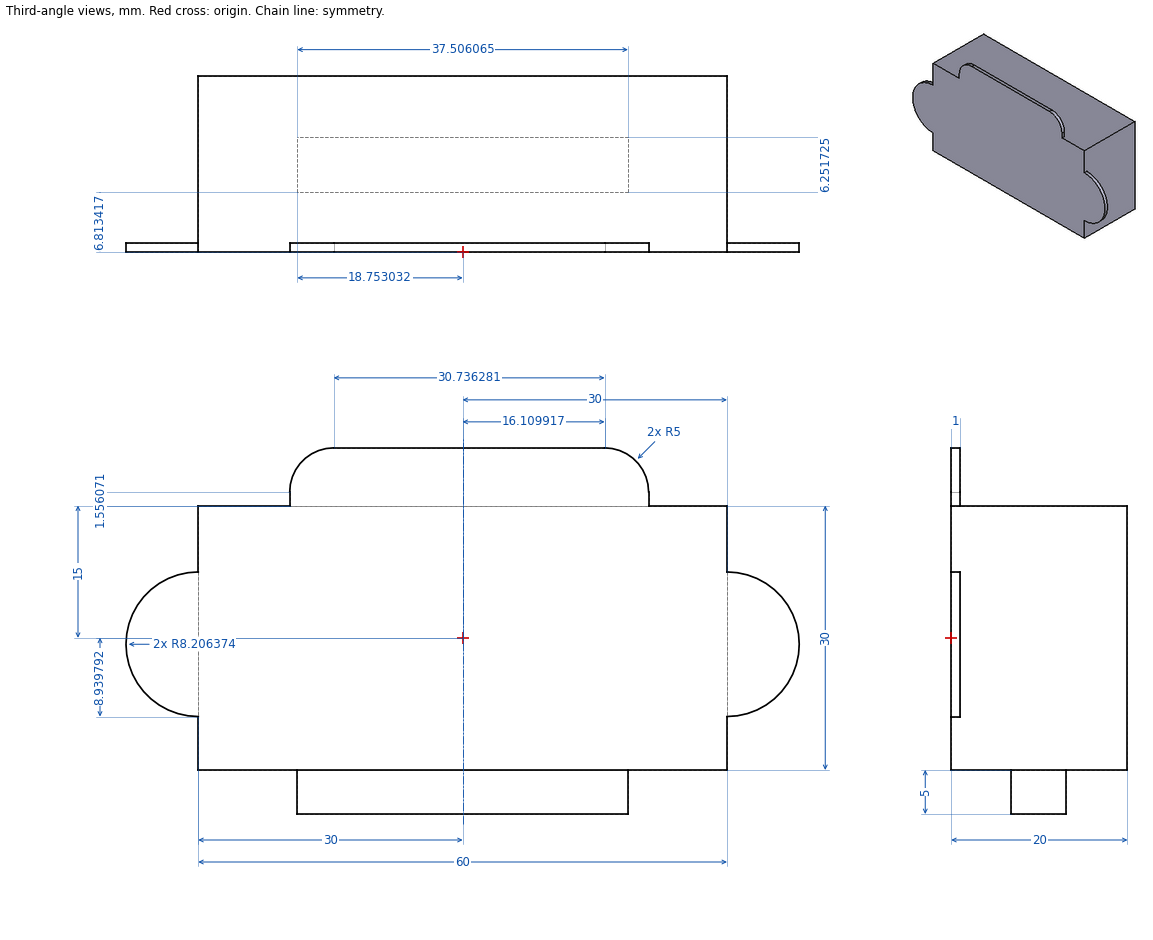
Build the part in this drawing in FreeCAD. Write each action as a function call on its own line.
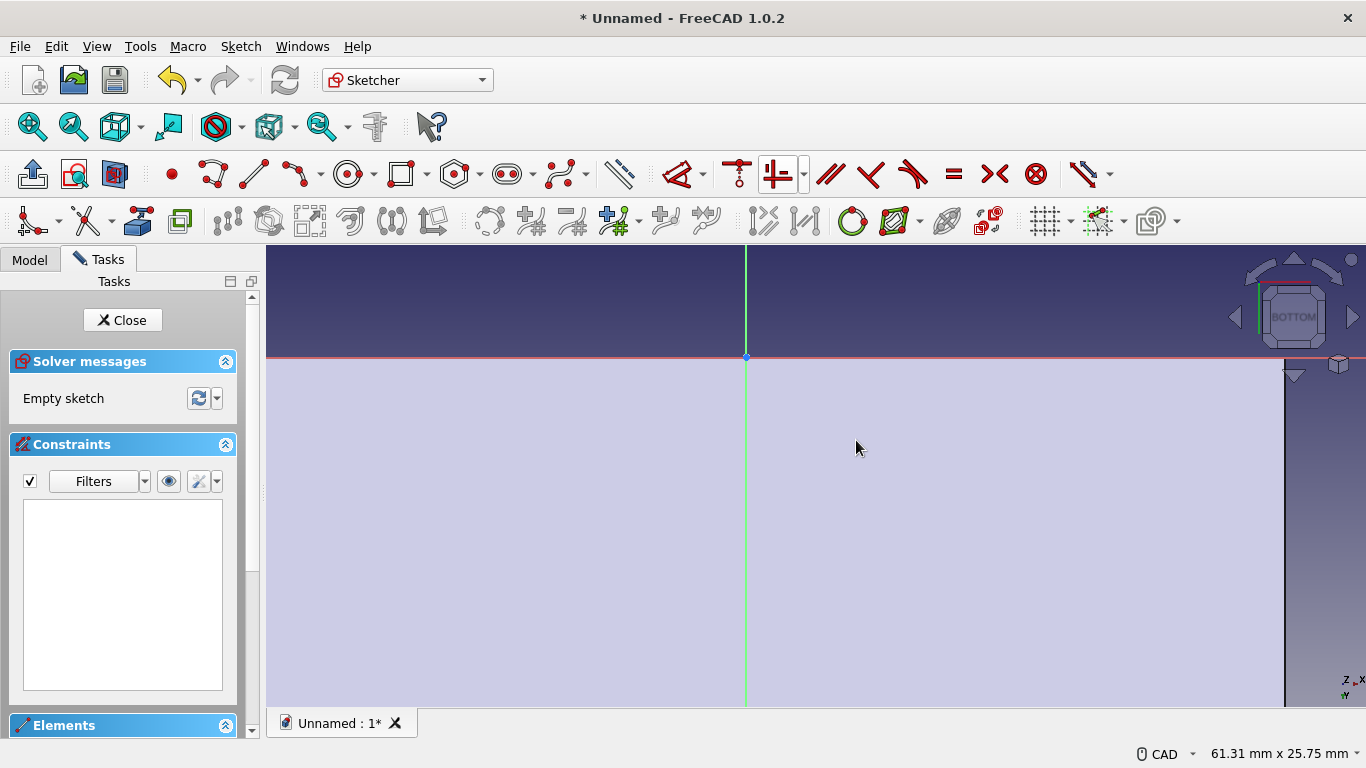
key(g)
key(r)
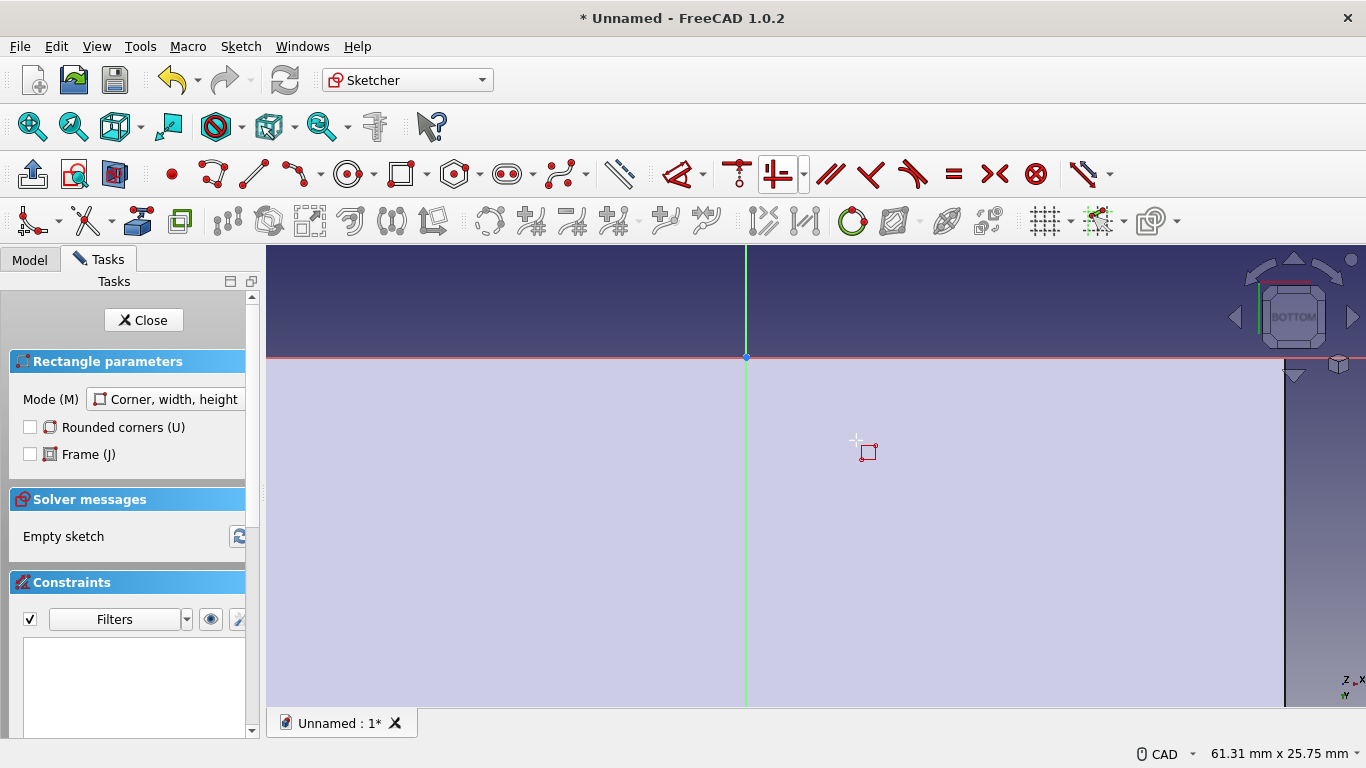
click(410, 480)
move(1083, 592)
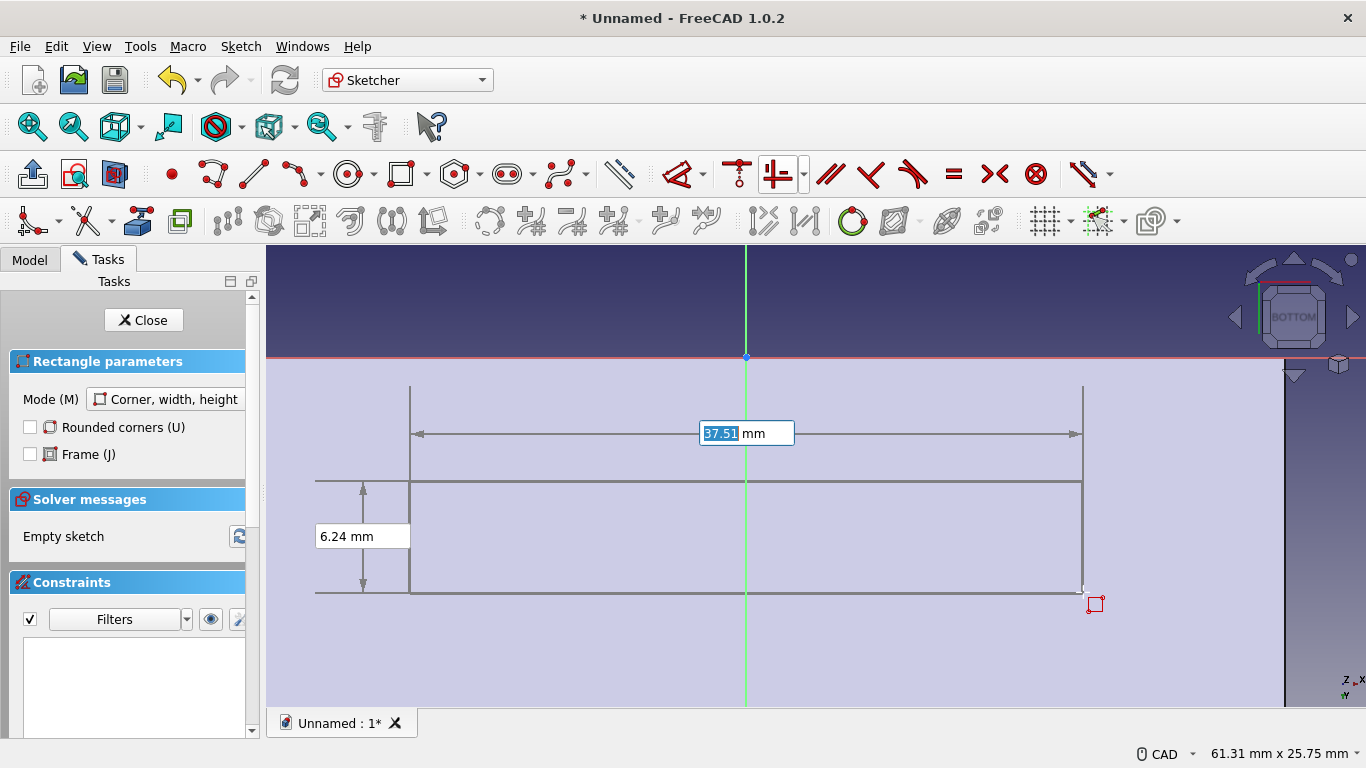
text(37.506065)
key(Tab)
text(6.251725)
key(Return)
key(Escape)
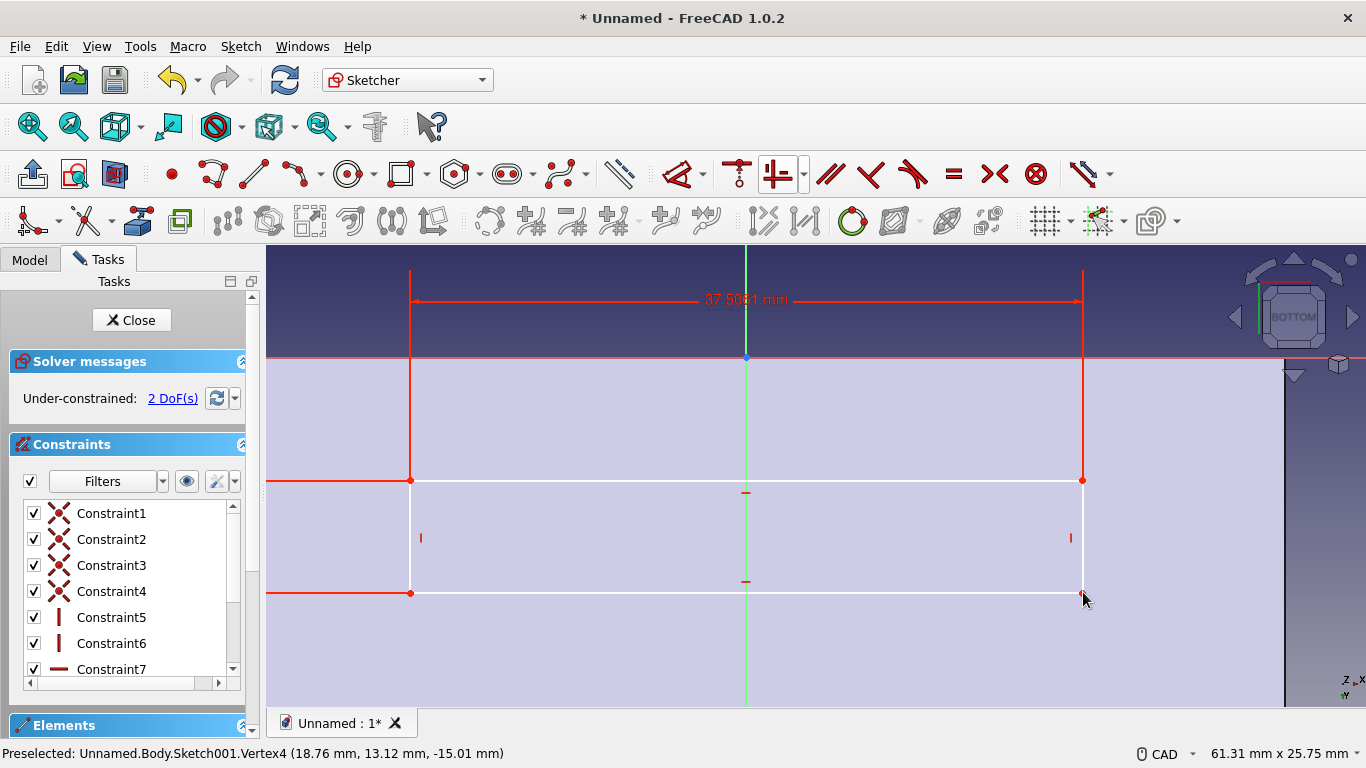
key(d)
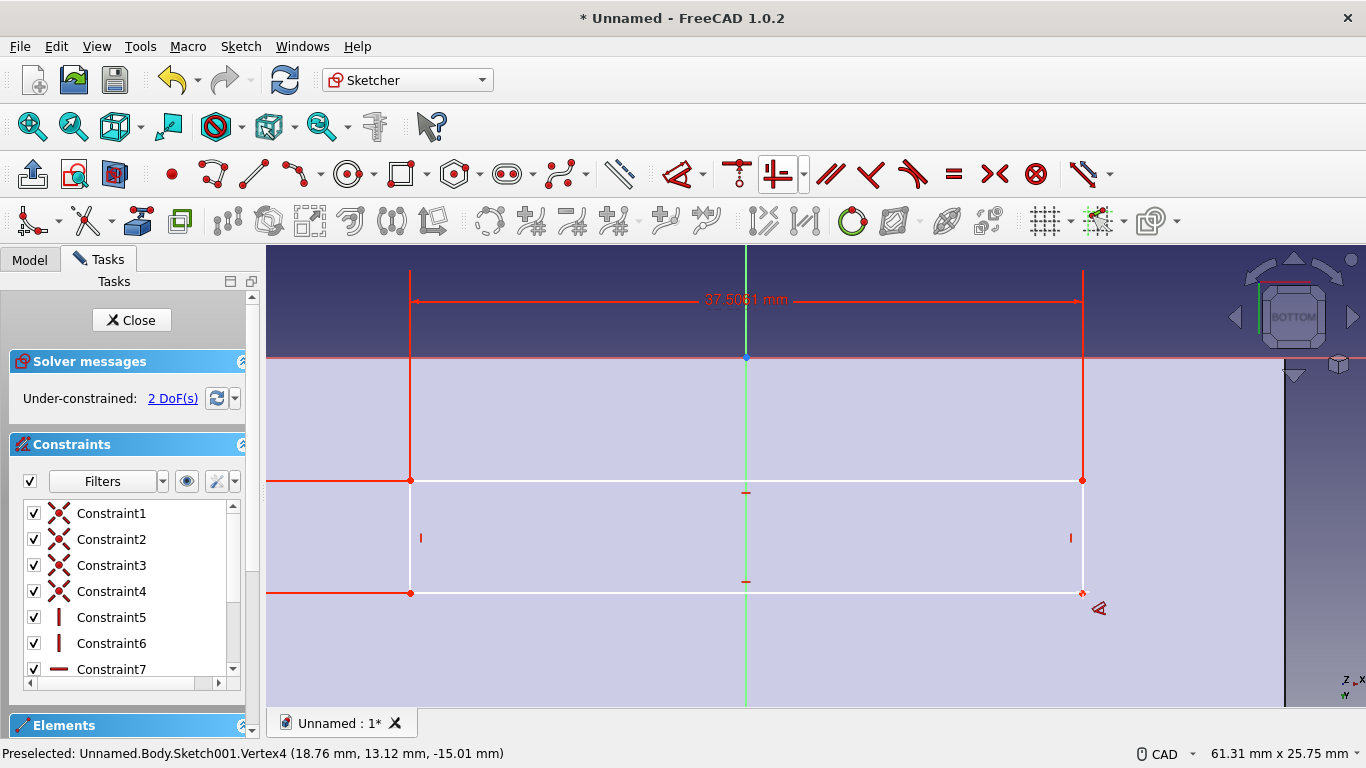
click(410, 481)
click(376, 419)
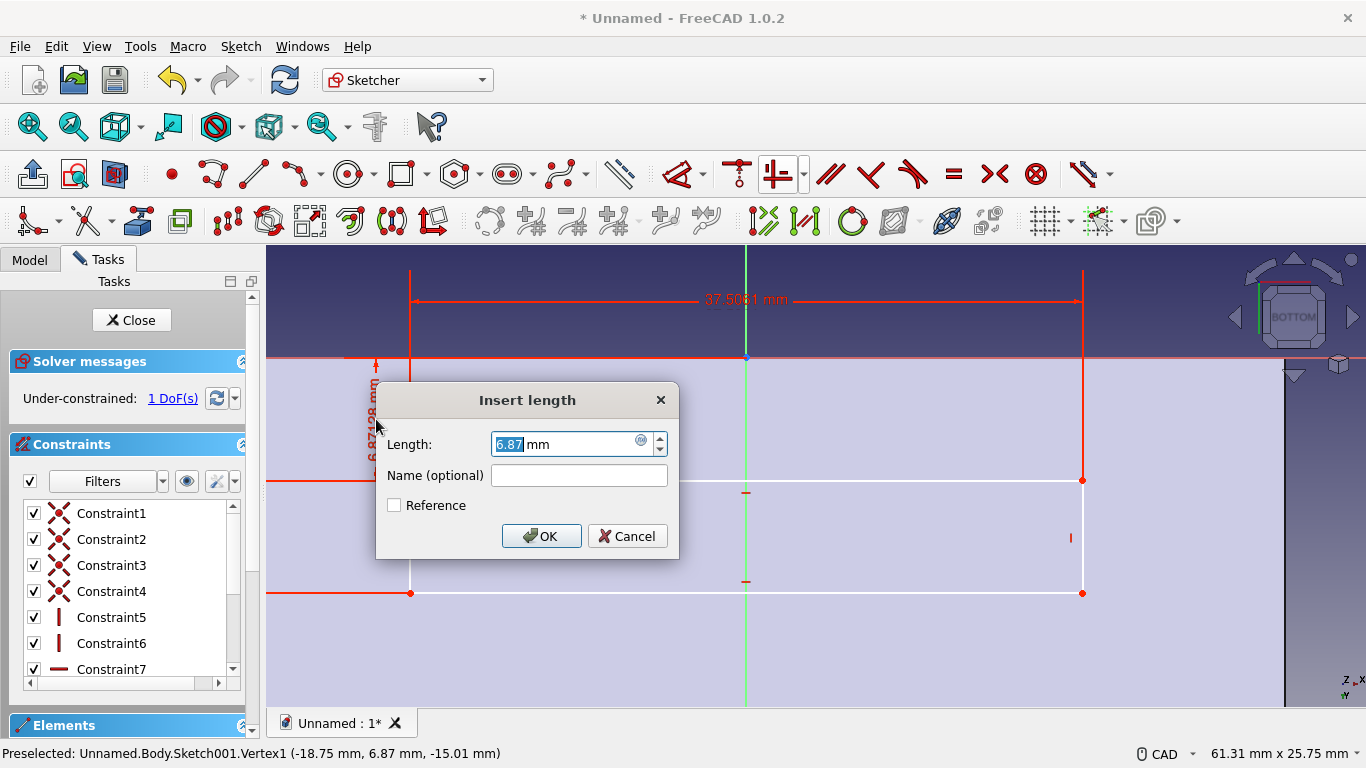
text(6.813417)
key(Return)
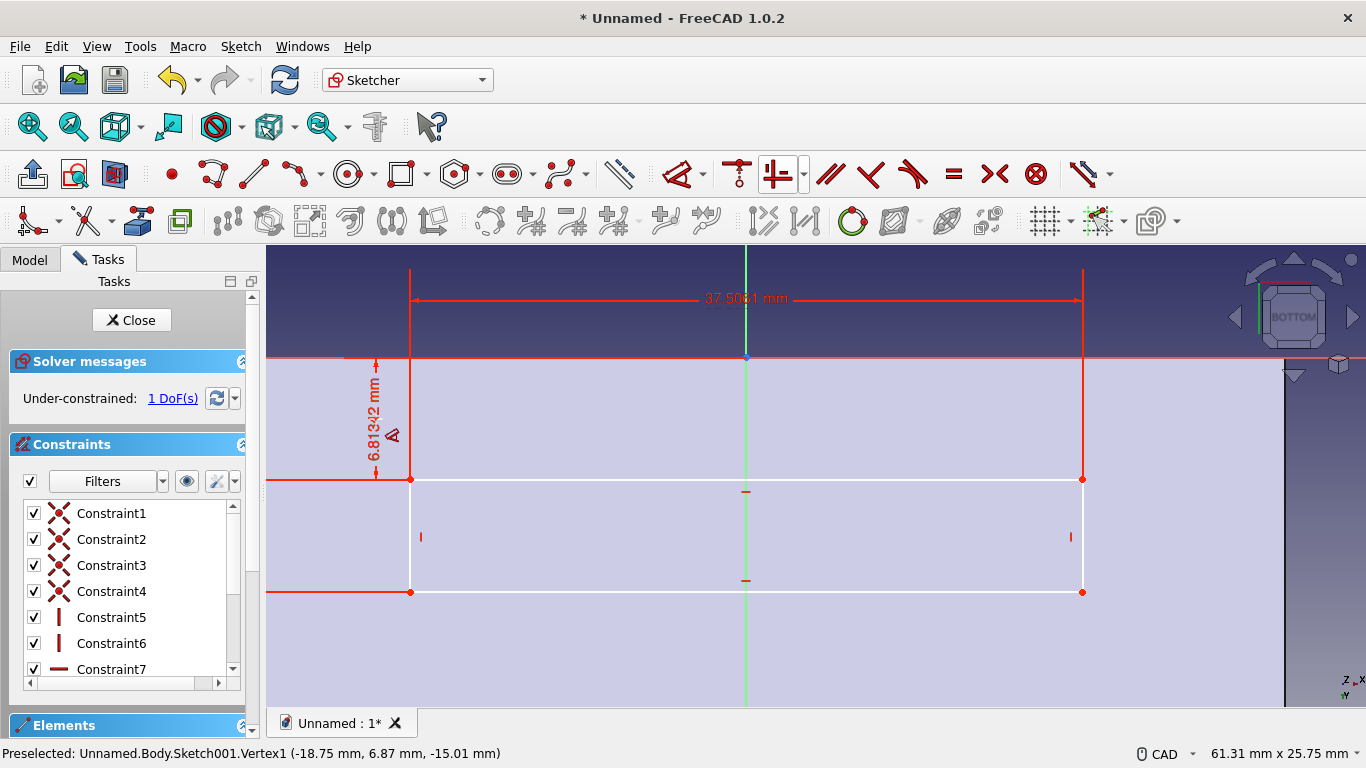
click(410, 480)
click(578, 324)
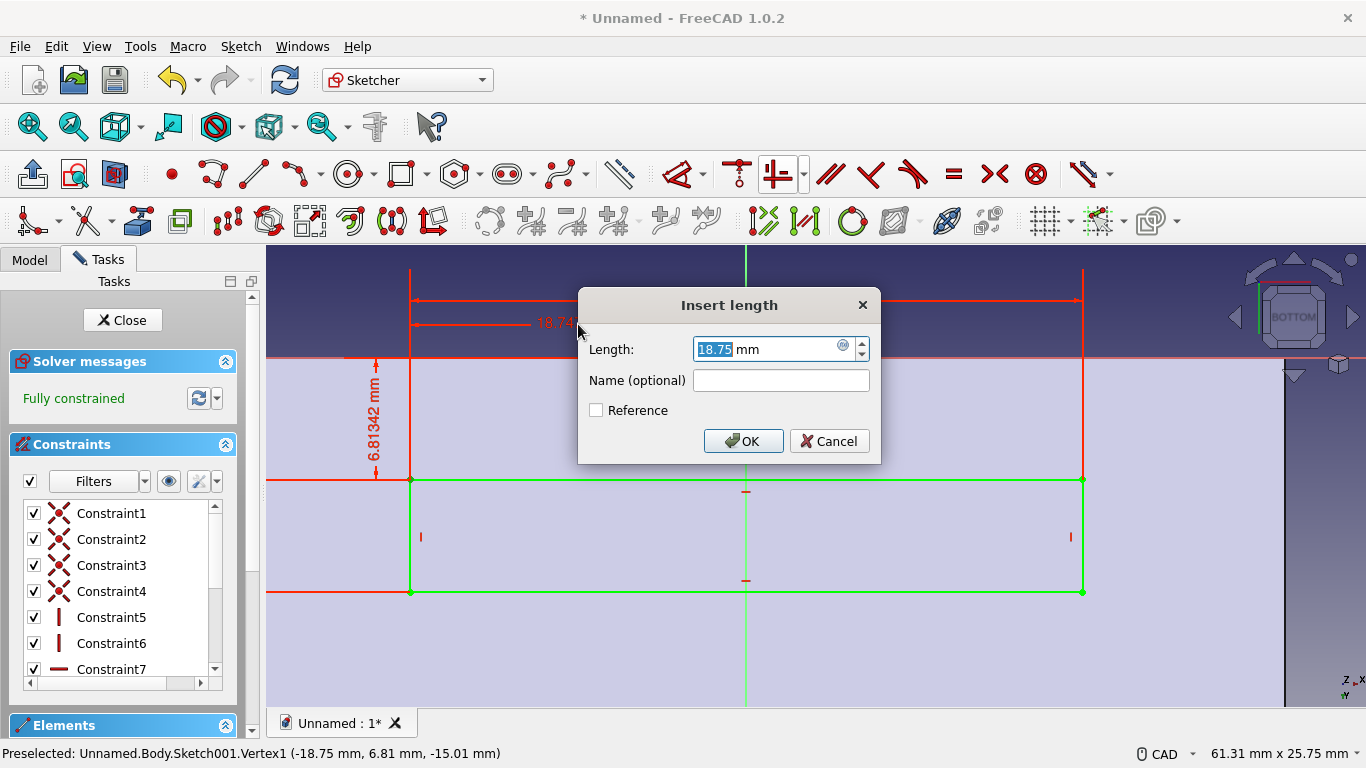
text(18.753032)
key(Return)
key(Escape)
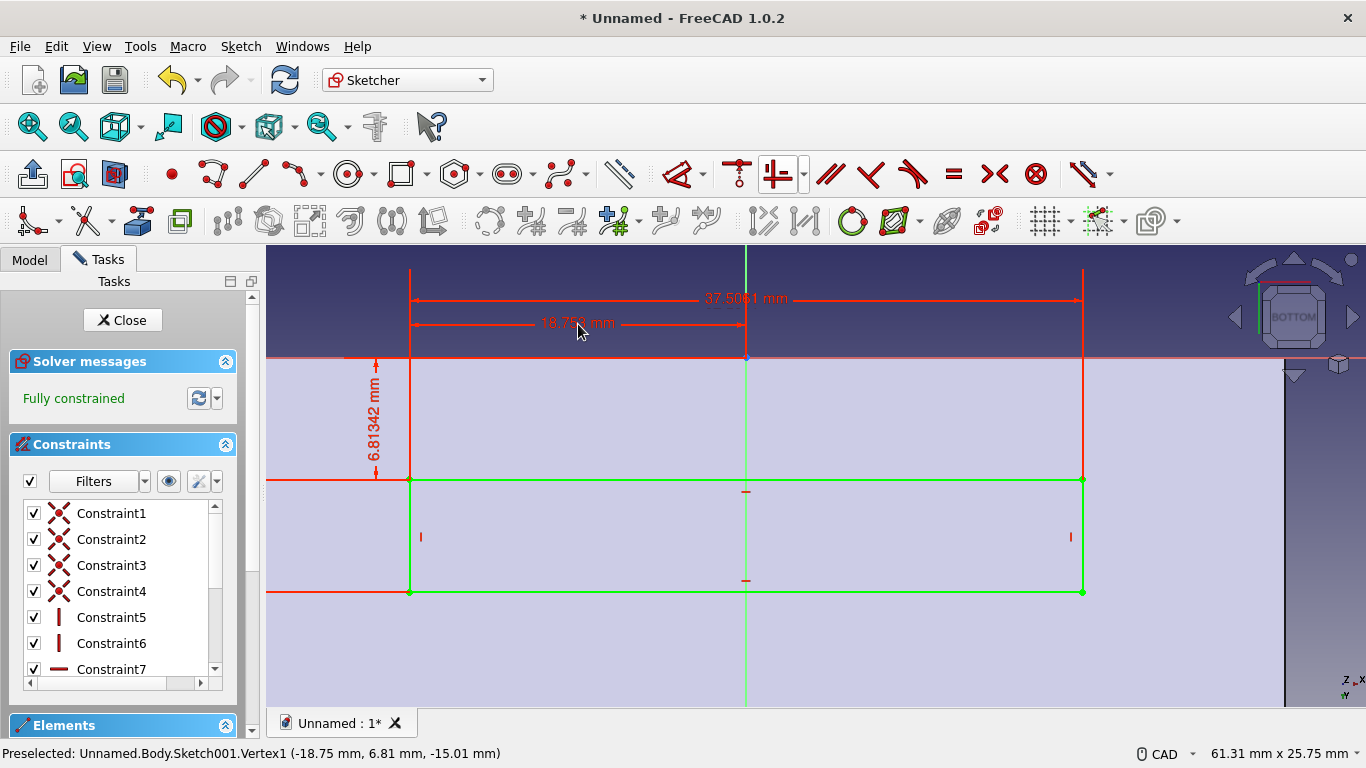
click(123, 320)